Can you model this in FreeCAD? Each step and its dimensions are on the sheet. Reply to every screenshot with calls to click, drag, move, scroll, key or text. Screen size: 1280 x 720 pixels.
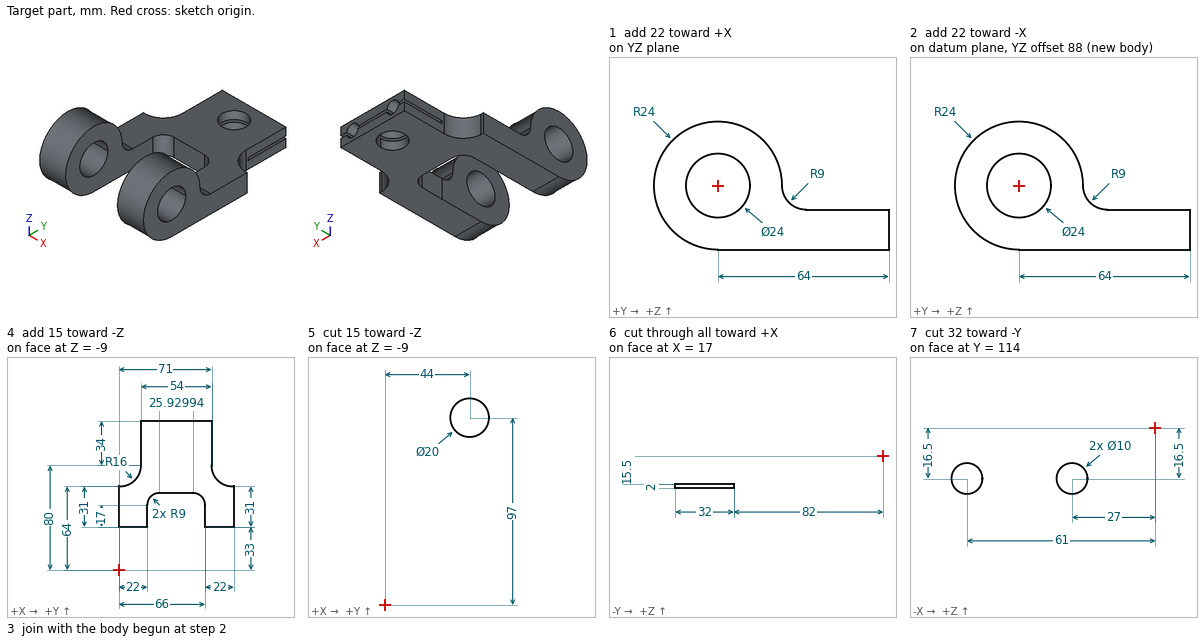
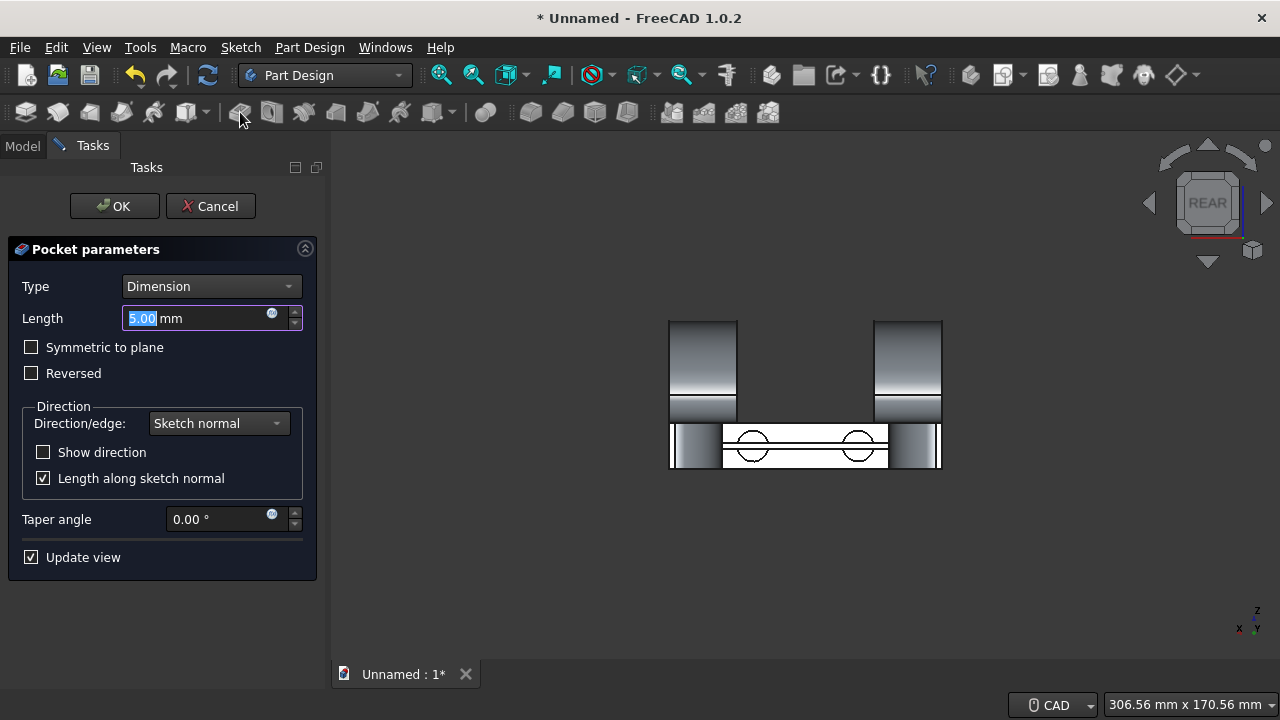
text(32)
key(Tab)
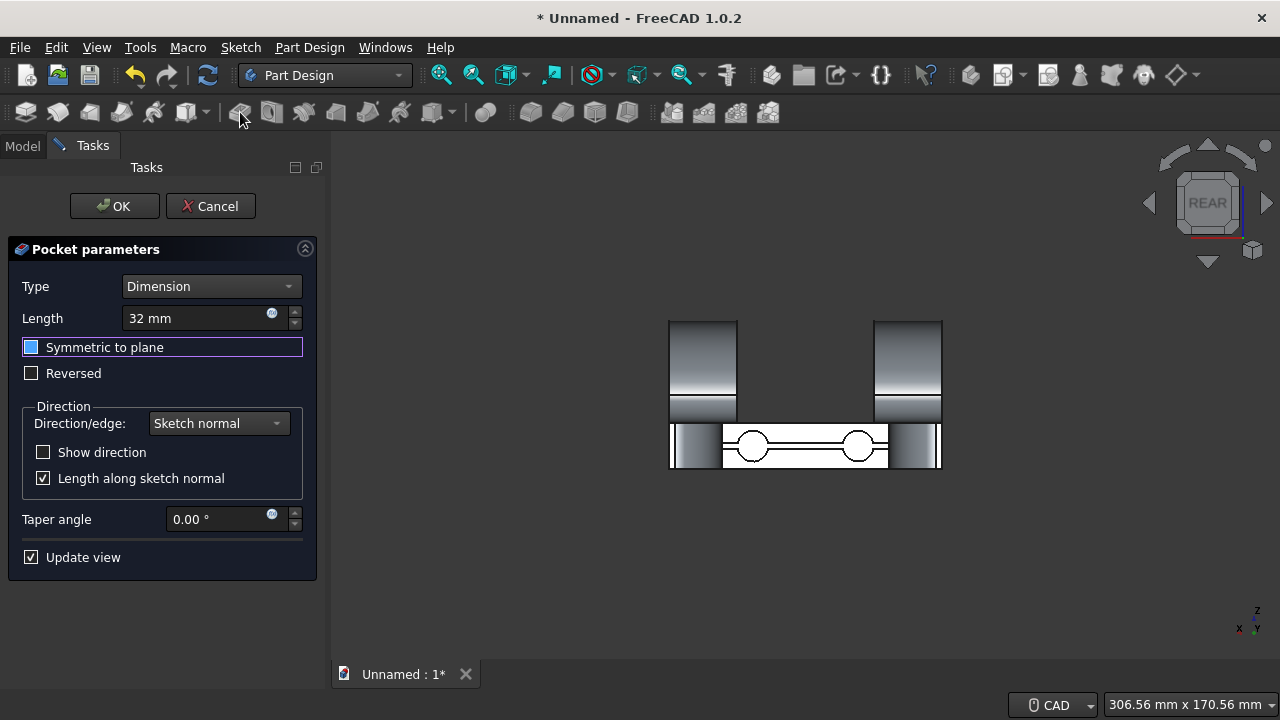
click(115, 206)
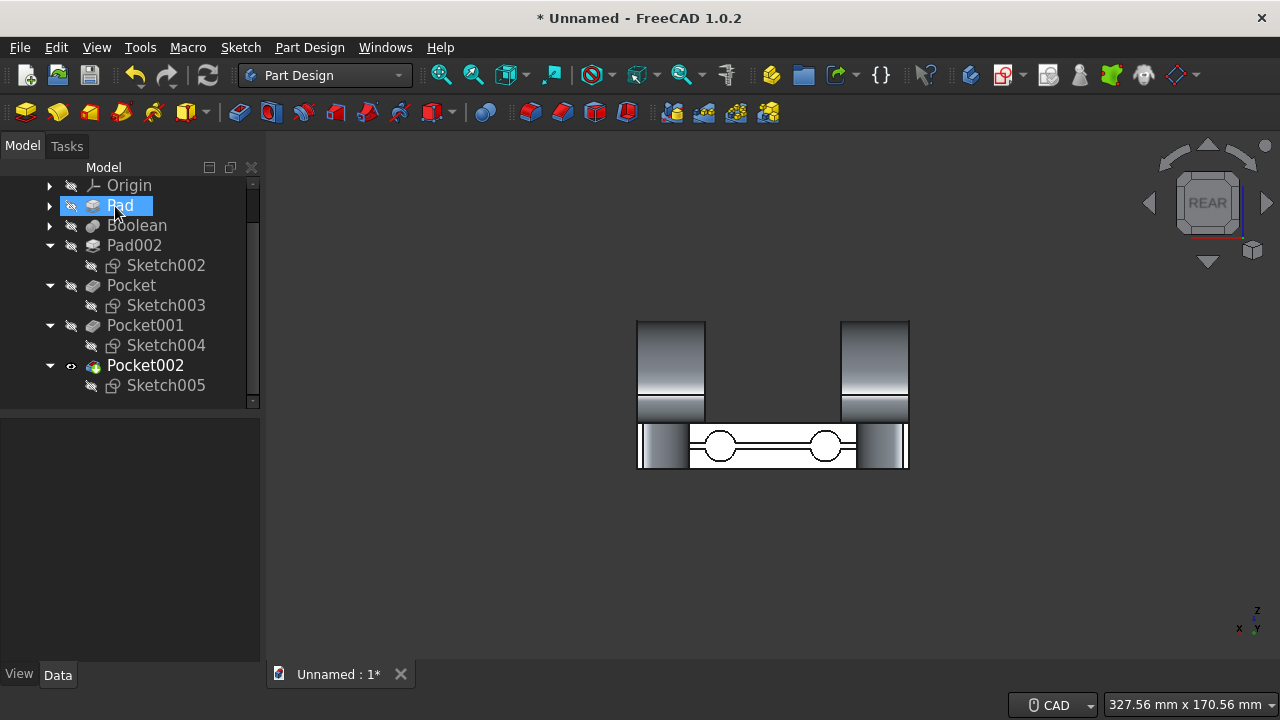
key(0)